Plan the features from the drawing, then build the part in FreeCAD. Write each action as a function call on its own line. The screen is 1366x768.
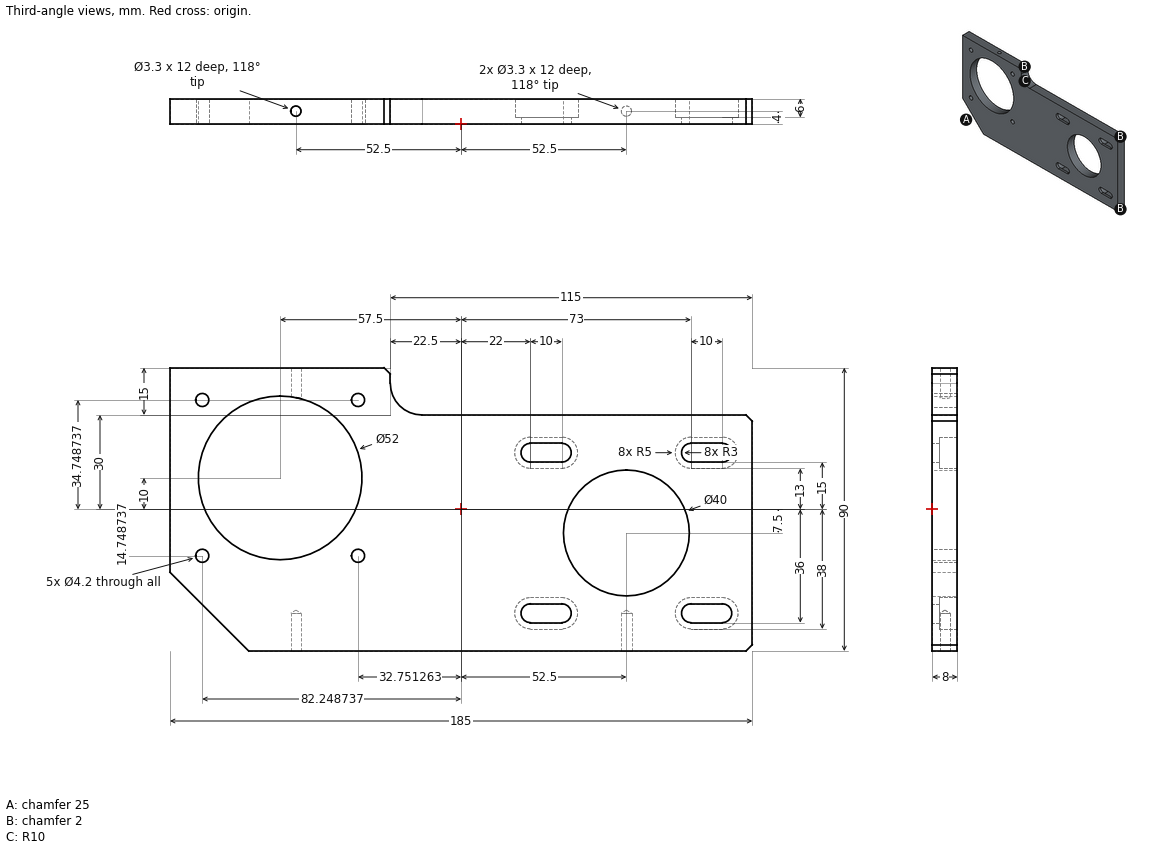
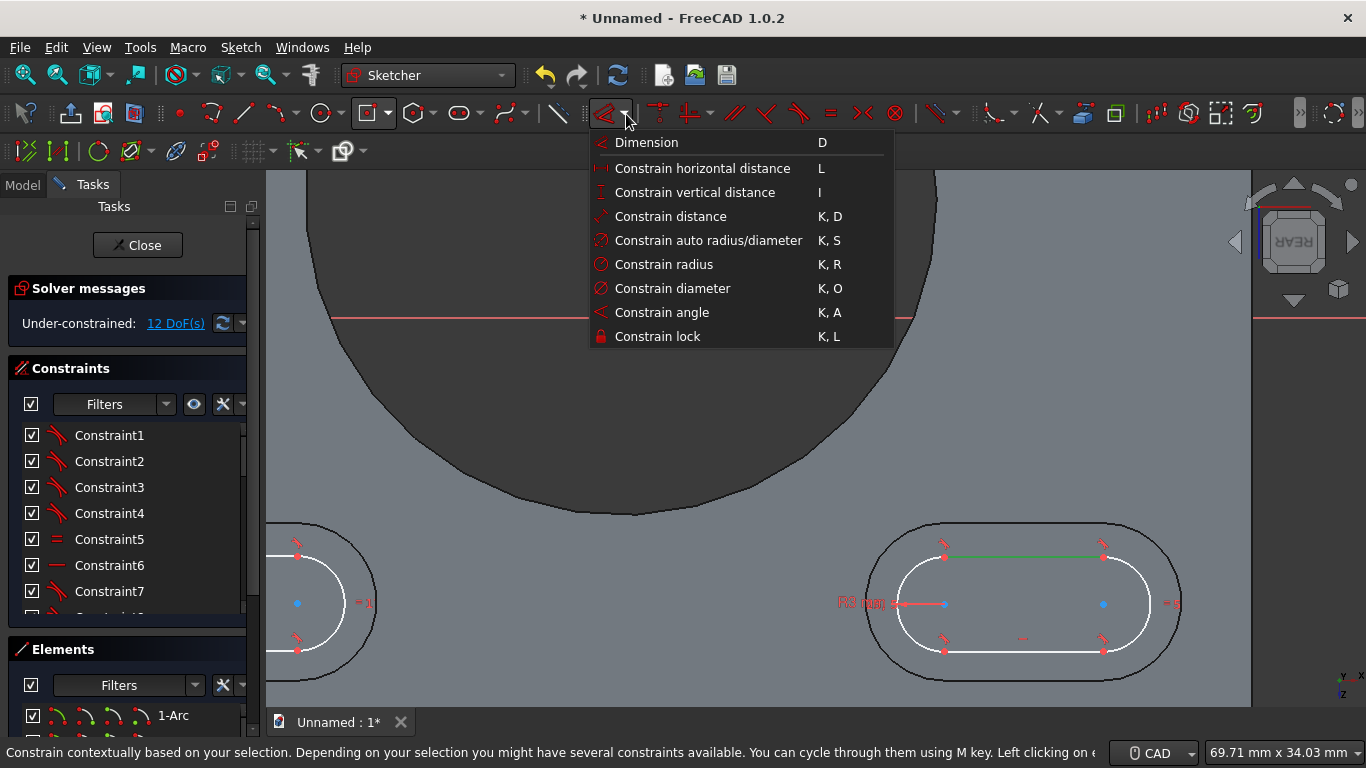
click(742, 168)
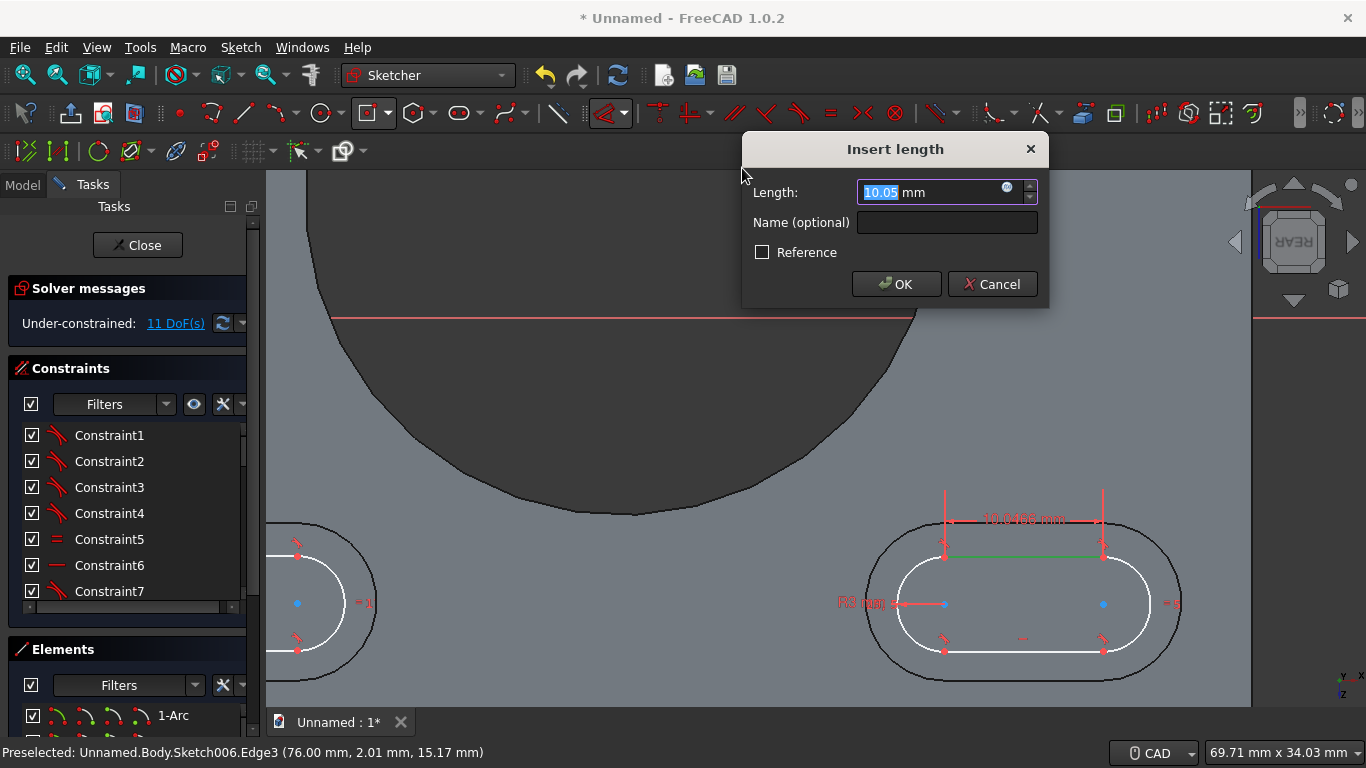
text(10)
key(Return)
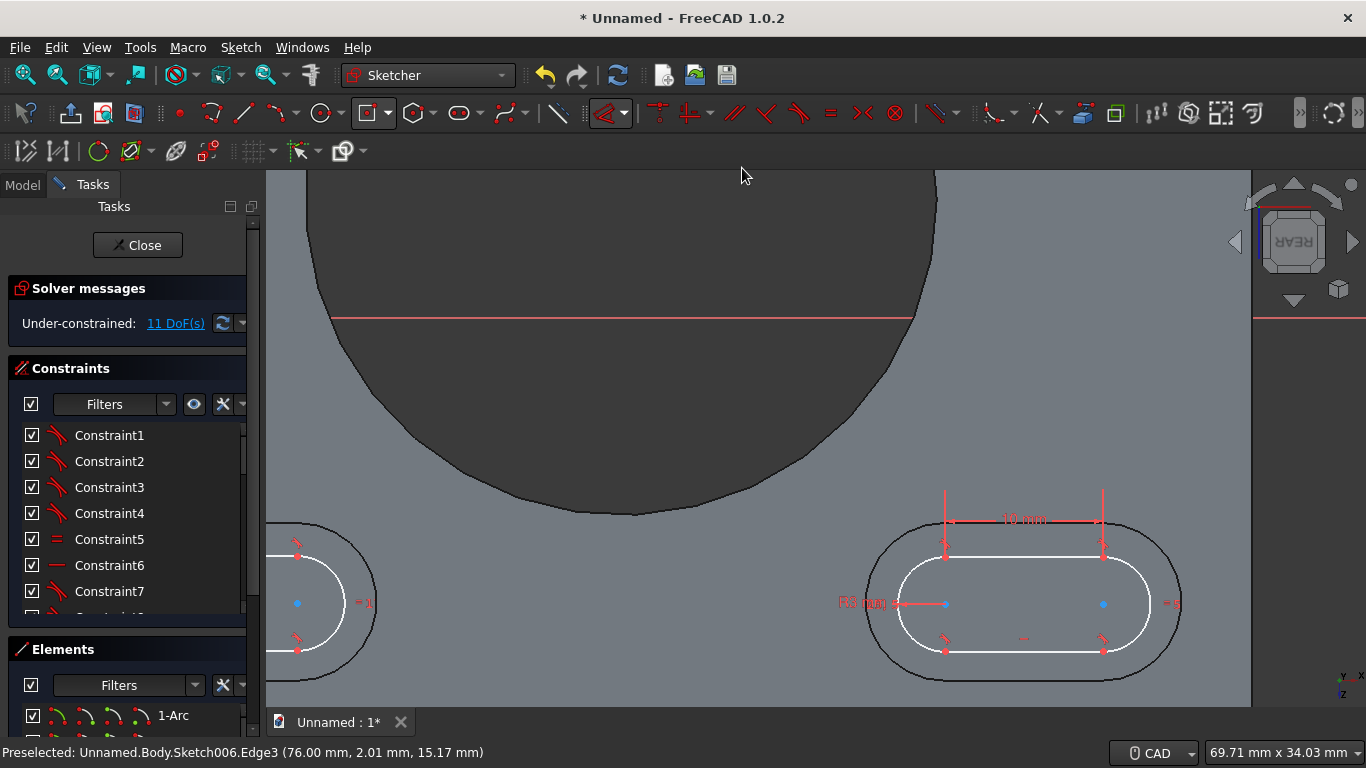
scroll(908, 578, down, 5)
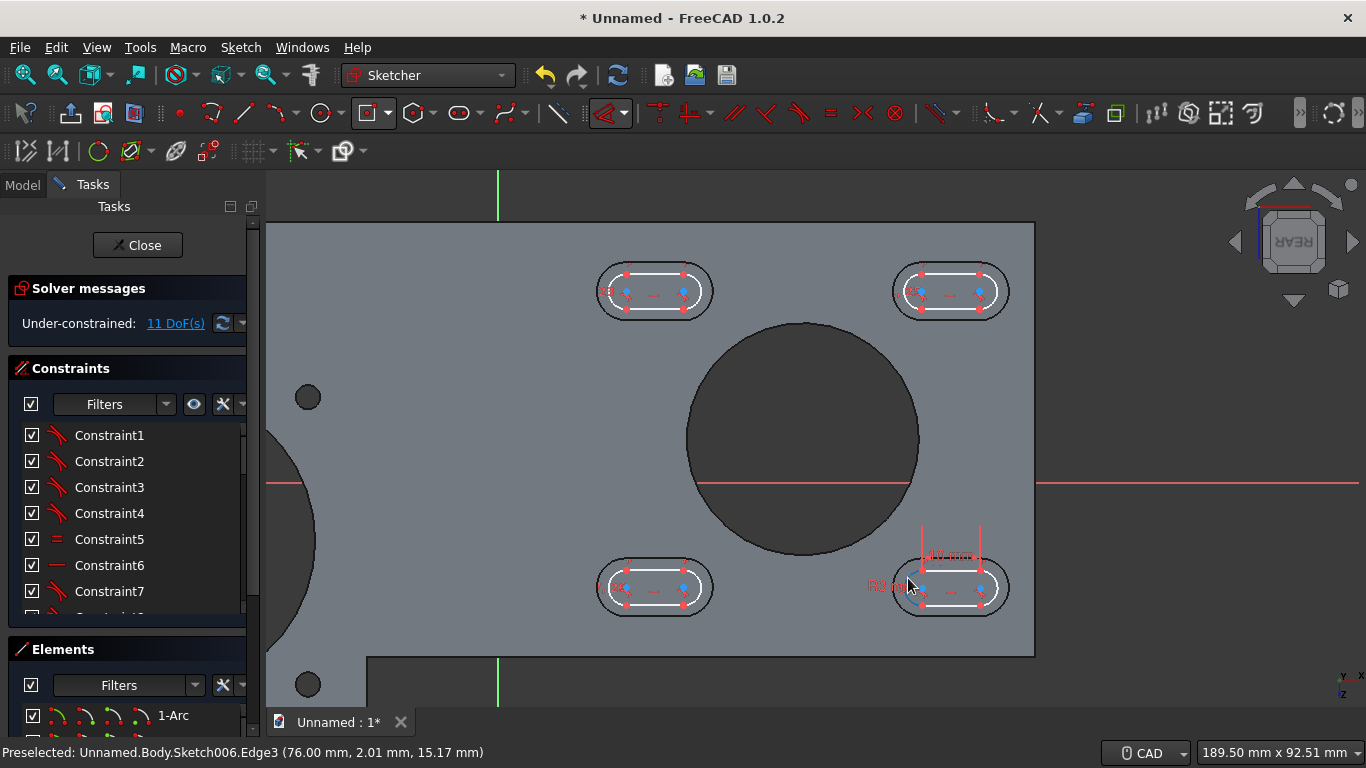
click(939, 274)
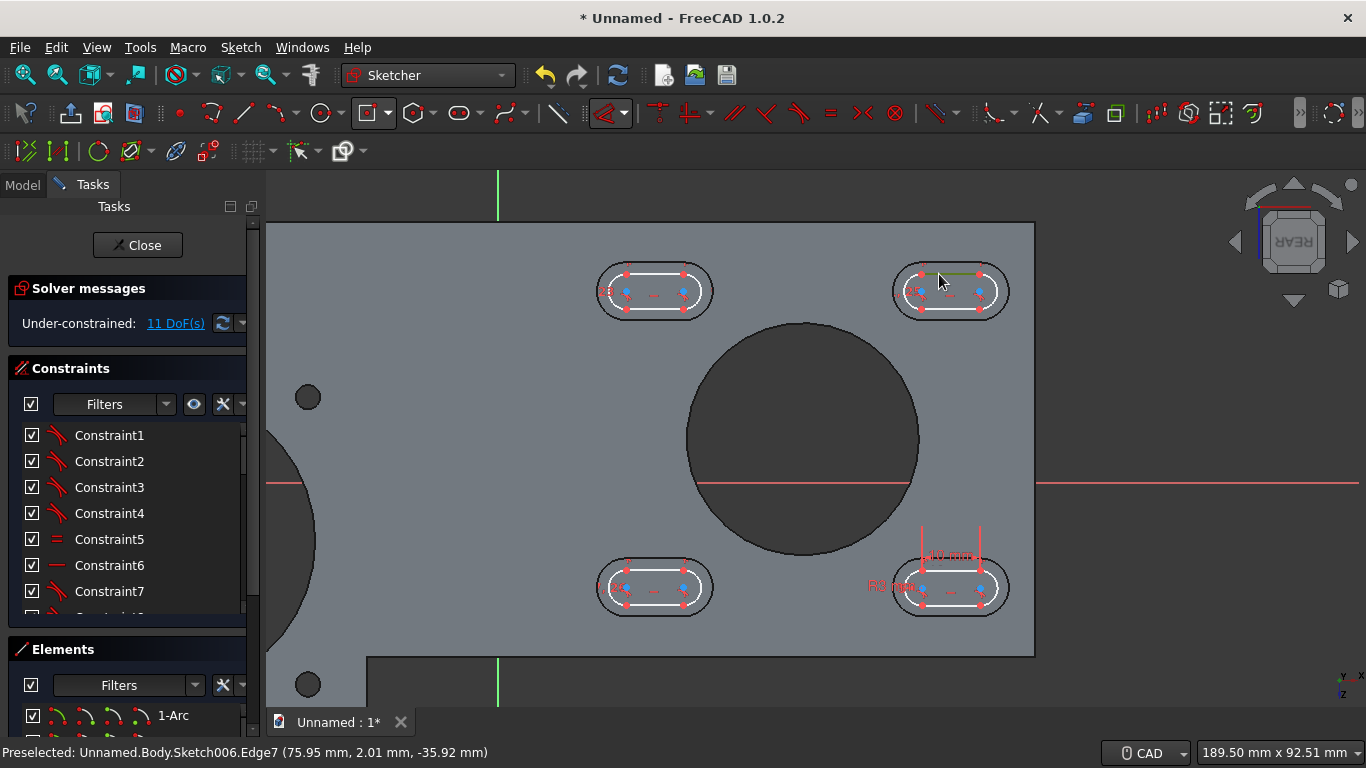
key(l)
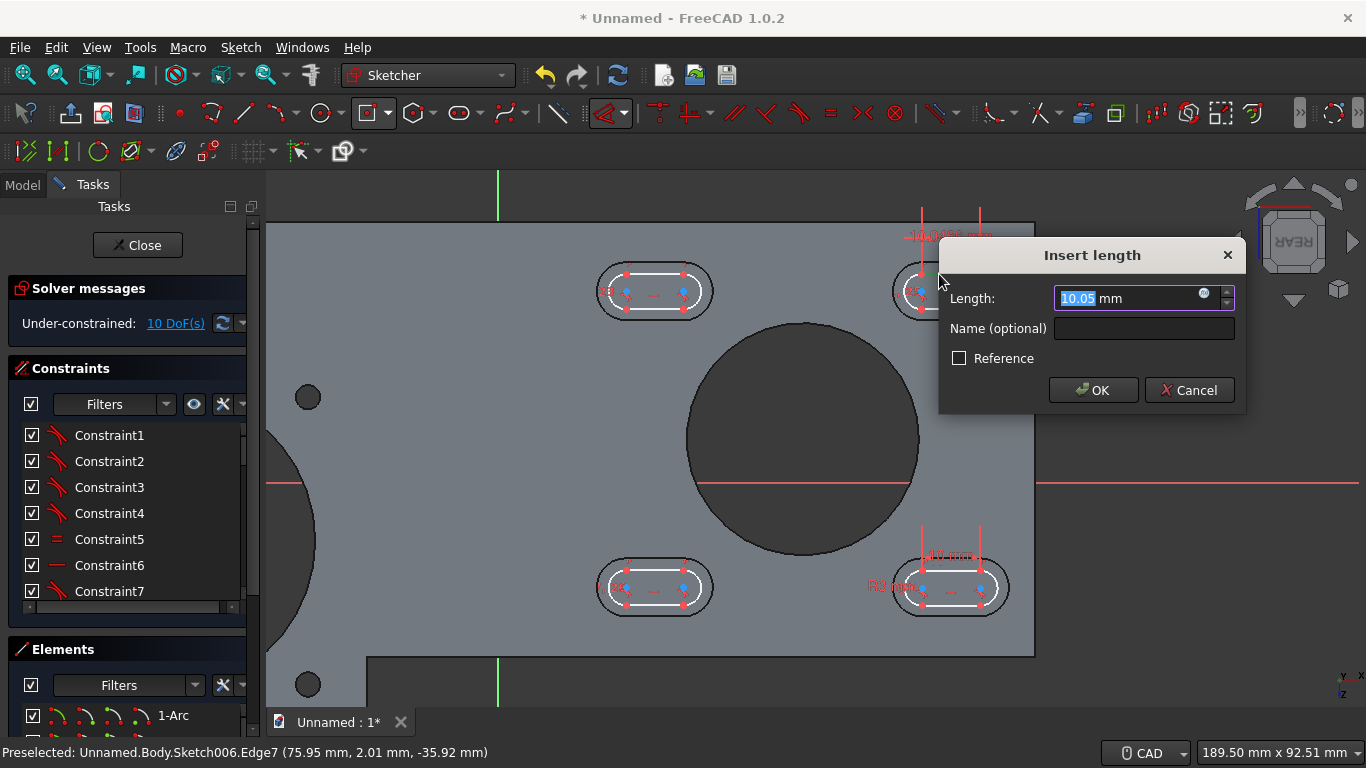
text(10)
key(Return)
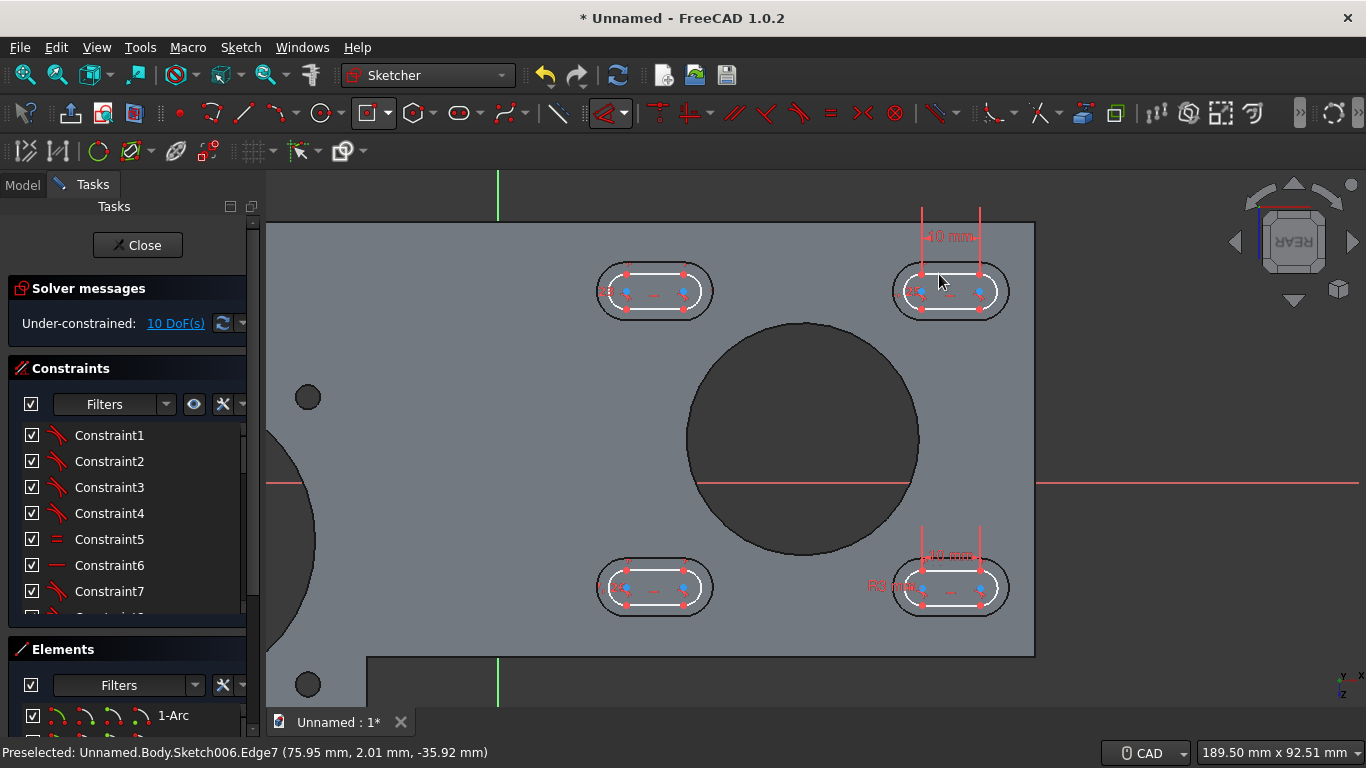
click(643, 570)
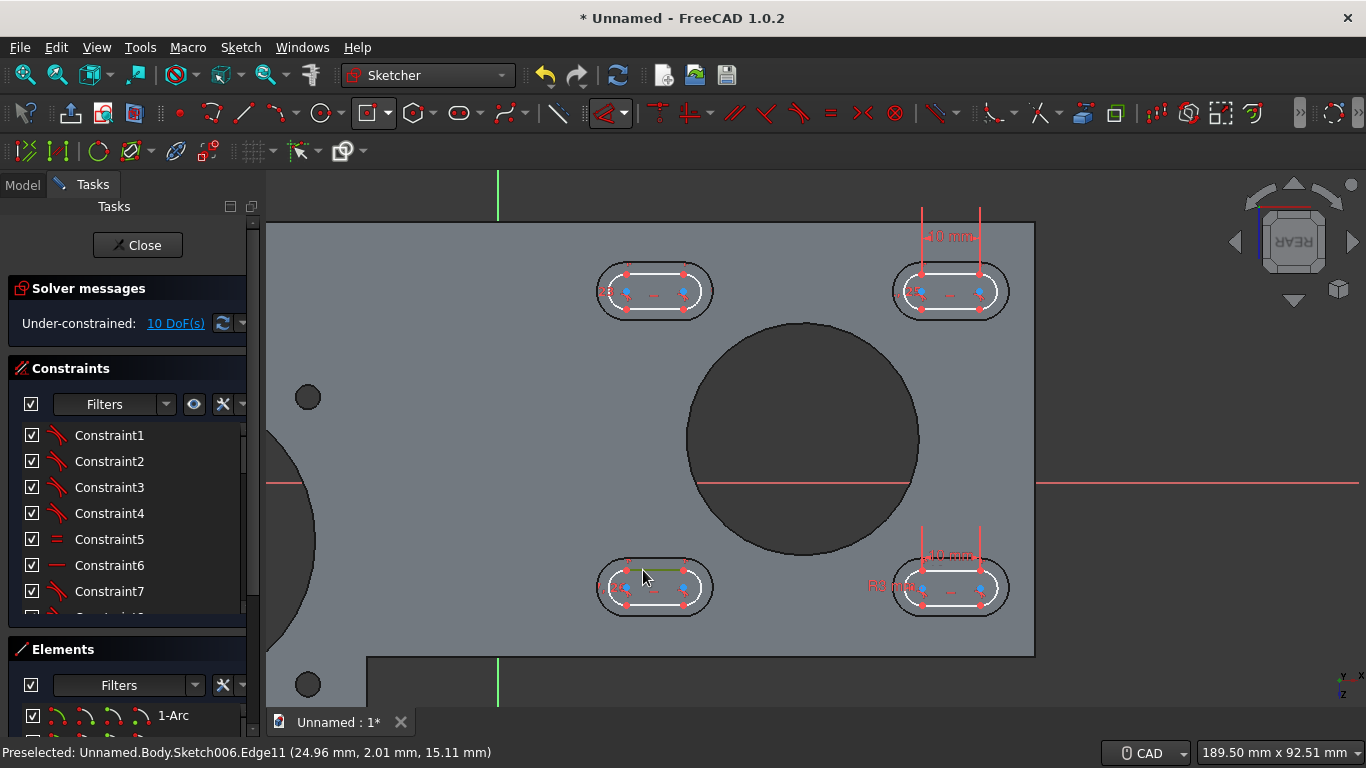
key(l)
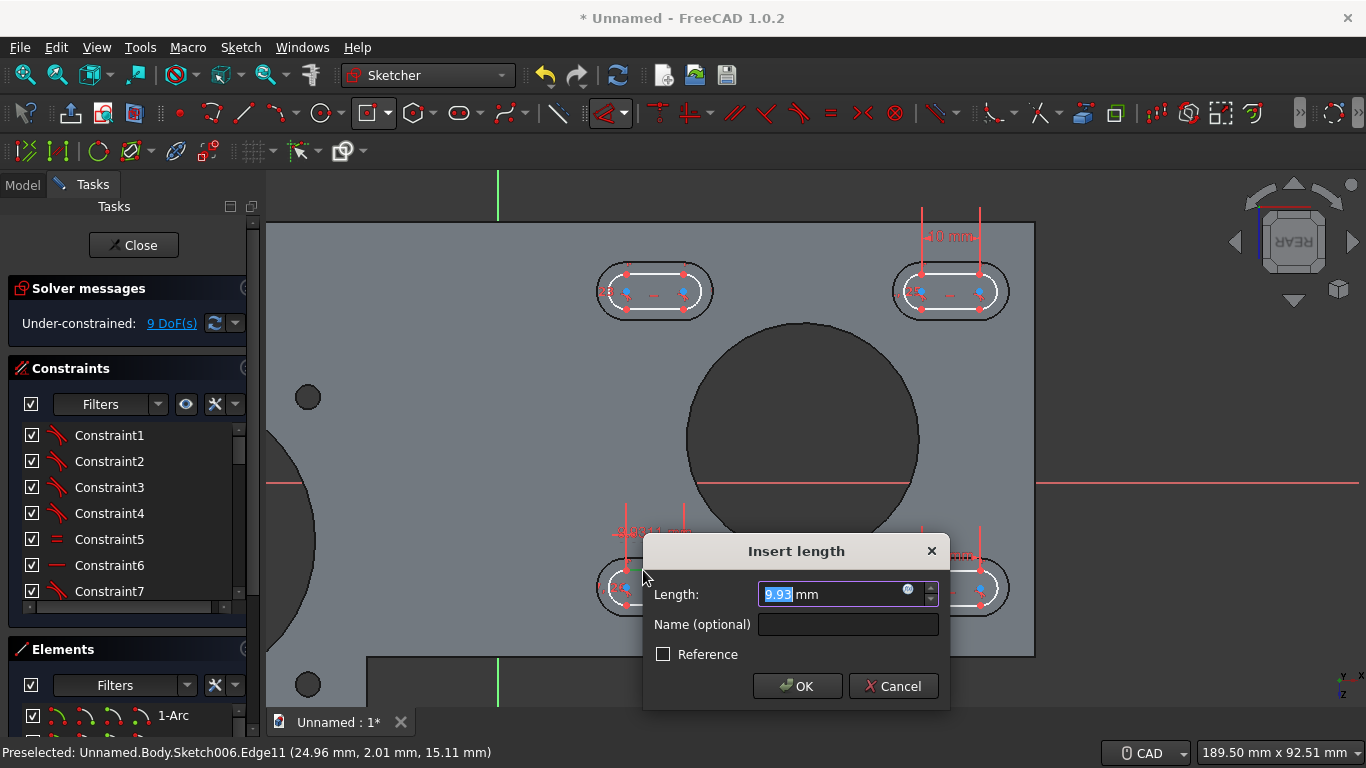
text(10)
key(Return)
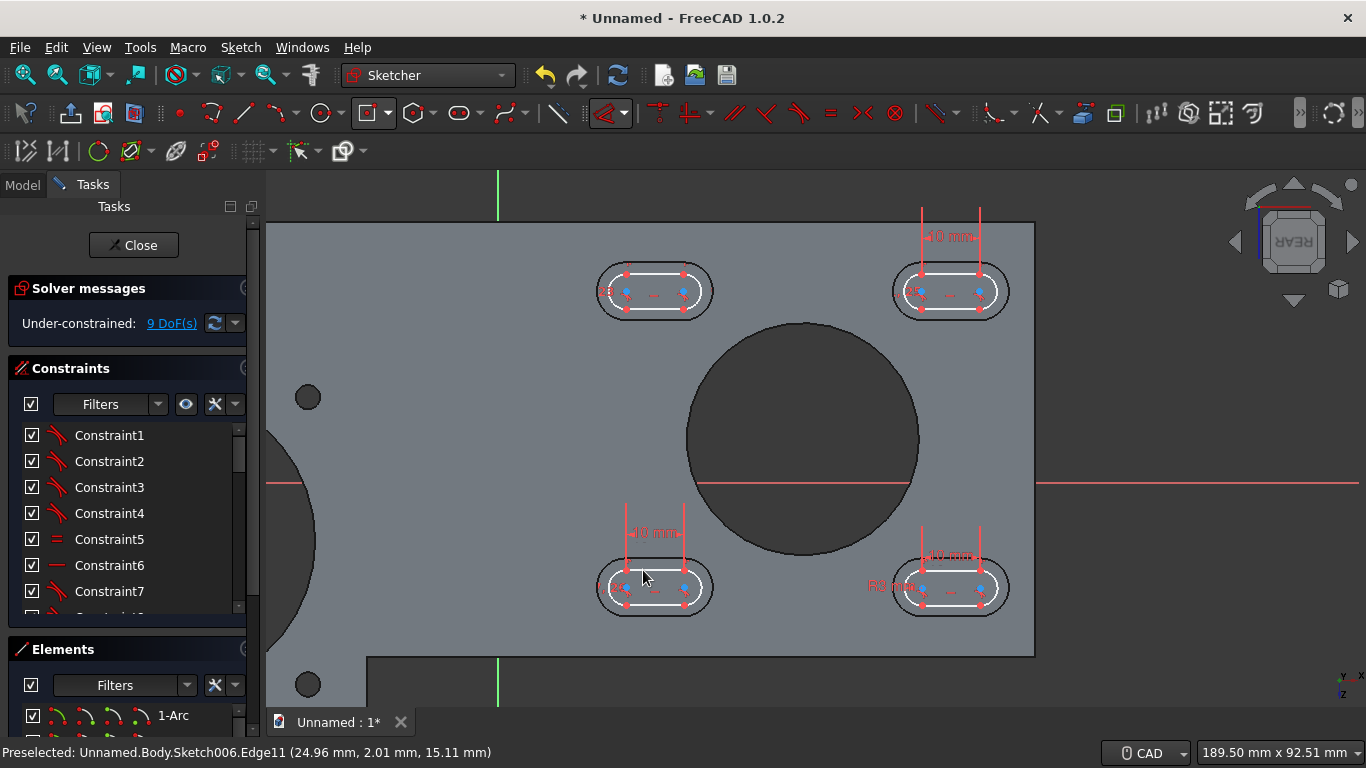
click(643, 274)